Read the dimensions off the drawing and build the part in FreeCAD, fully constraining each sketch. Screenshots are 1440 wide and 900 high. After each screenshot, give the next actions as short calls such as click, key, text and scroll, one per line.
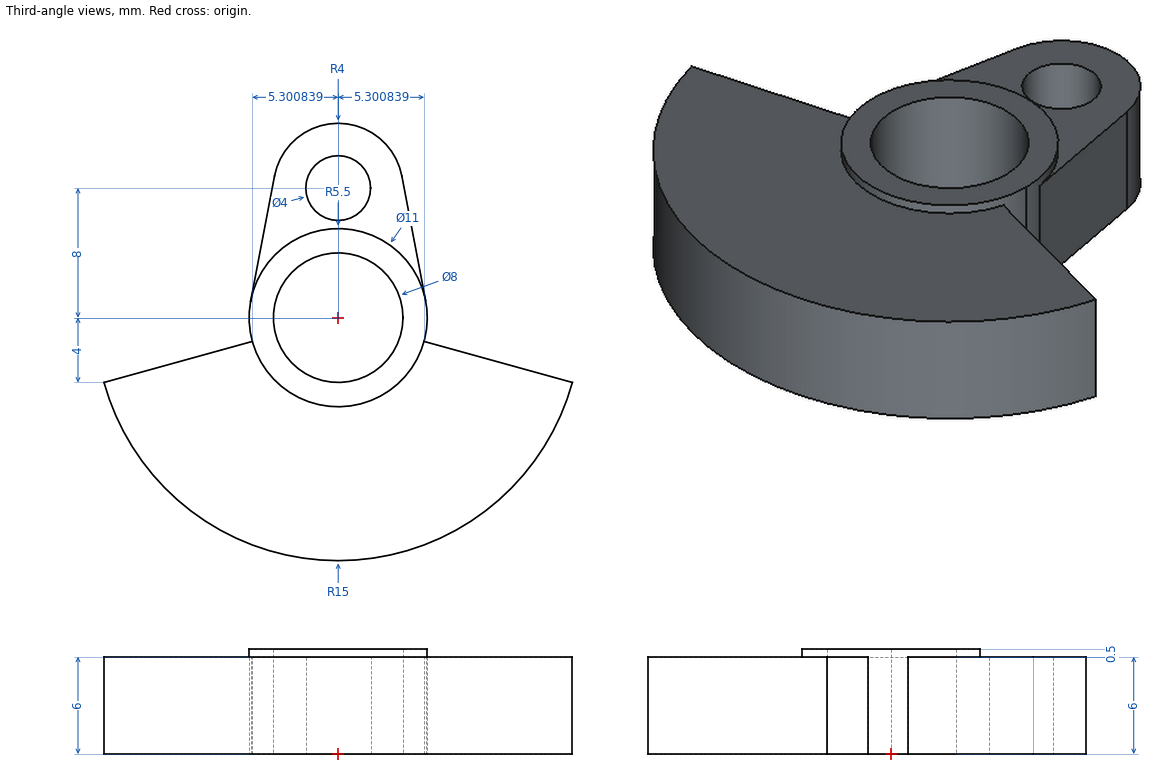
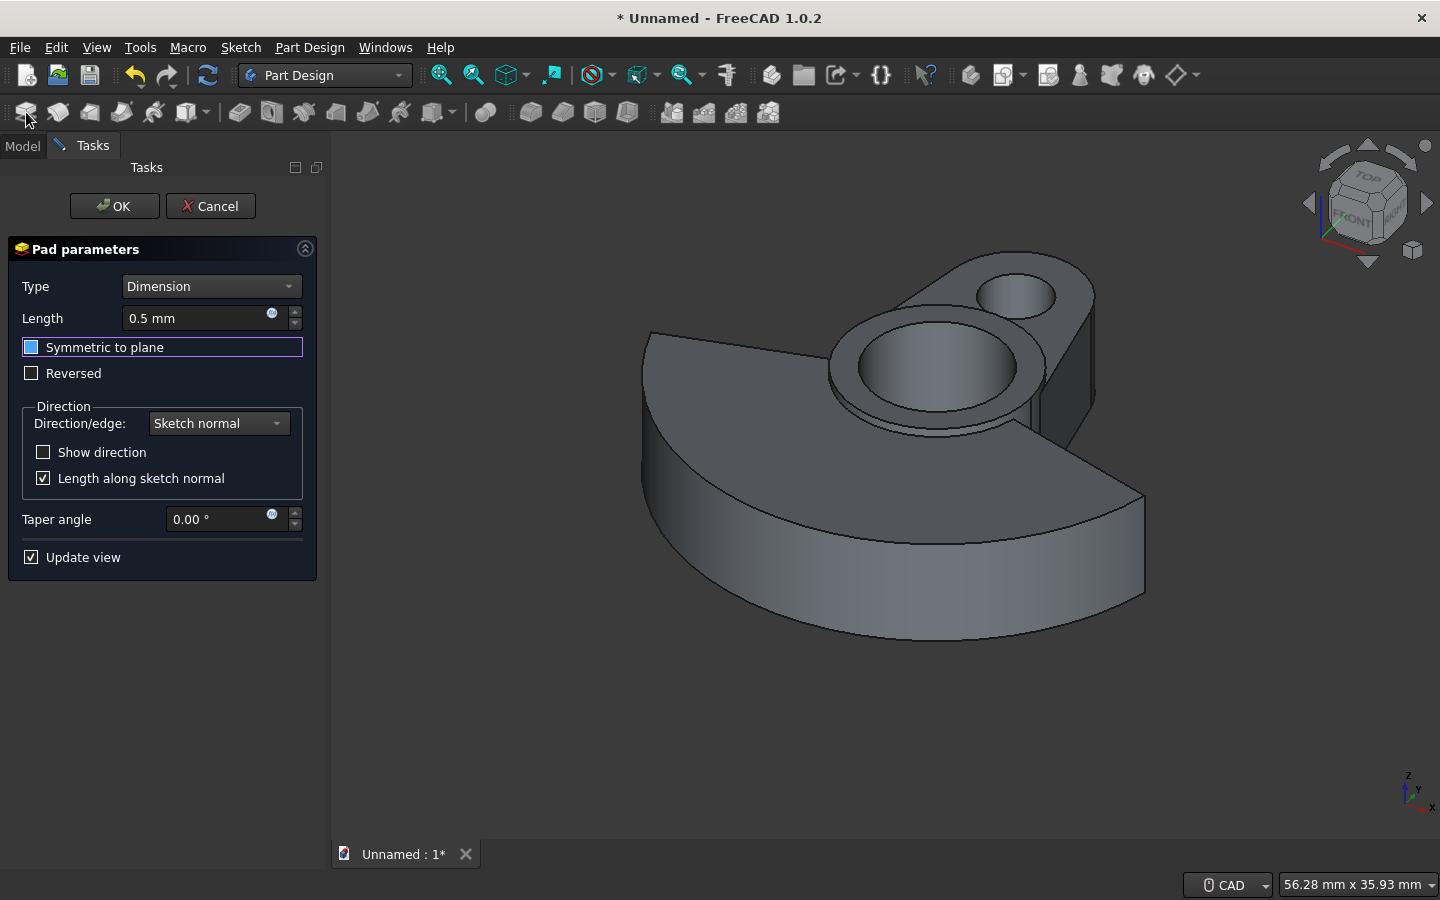
click(115, 206)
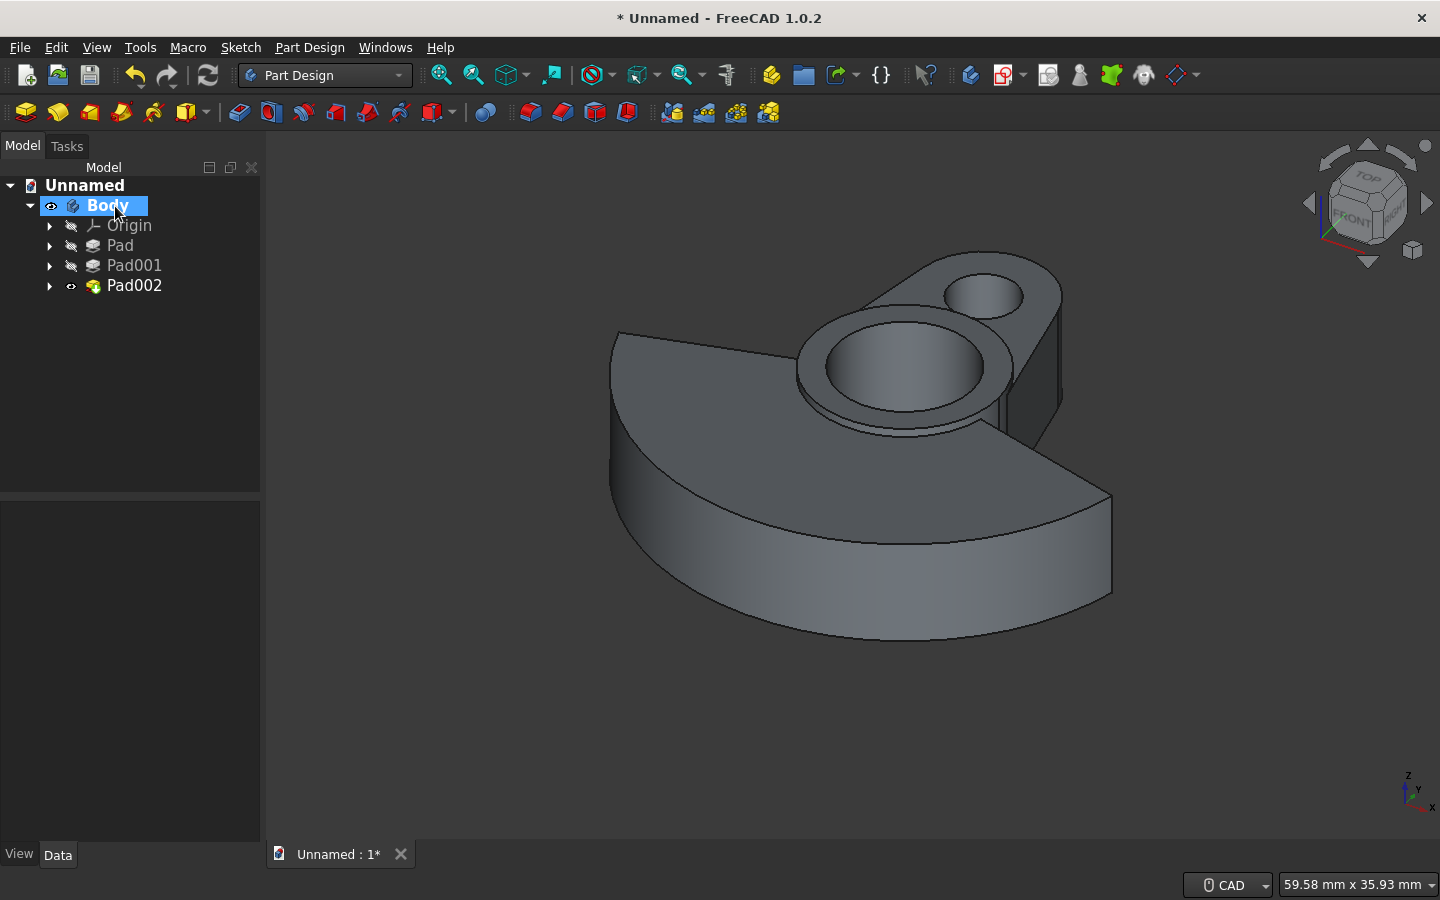
key(0)